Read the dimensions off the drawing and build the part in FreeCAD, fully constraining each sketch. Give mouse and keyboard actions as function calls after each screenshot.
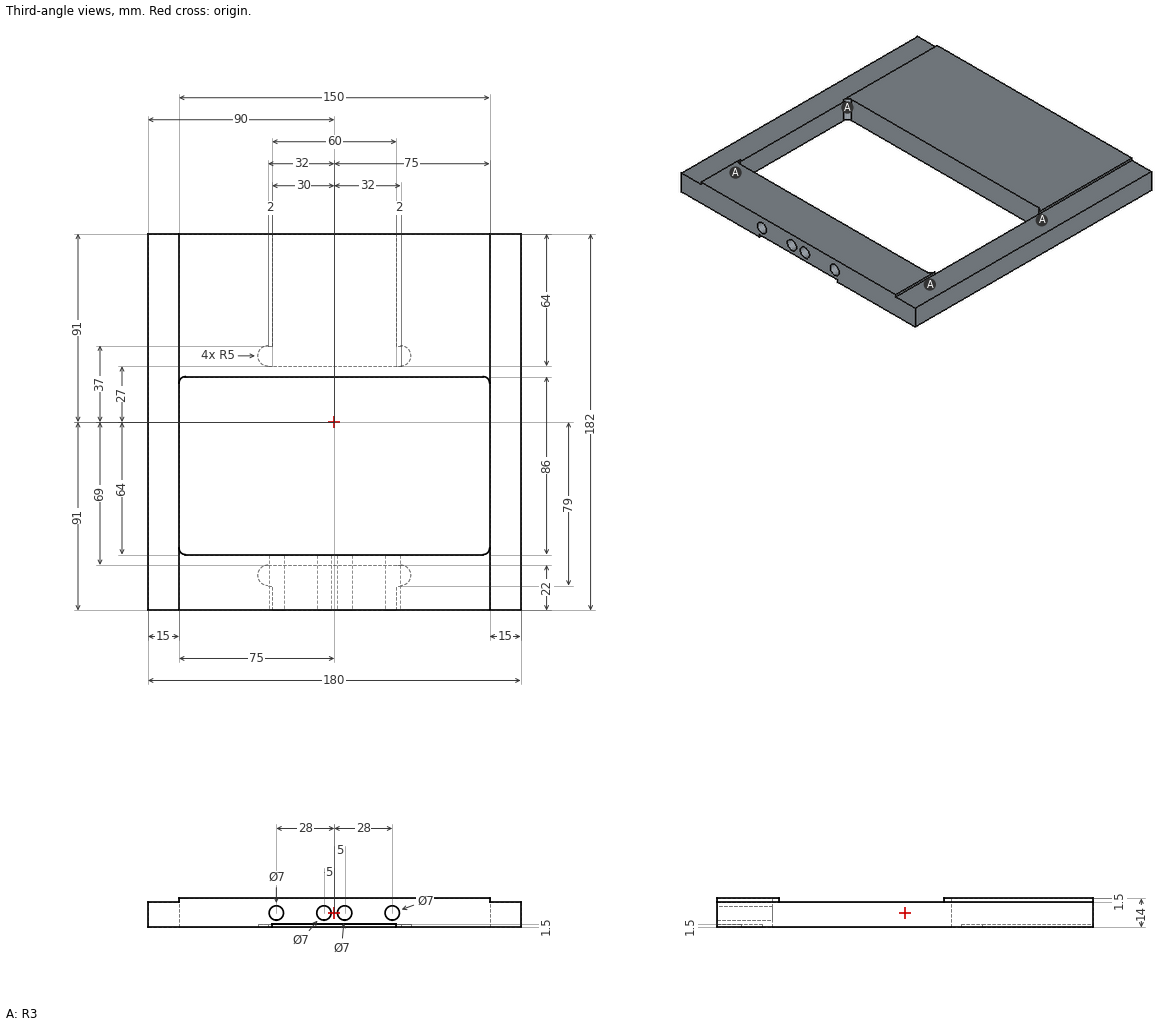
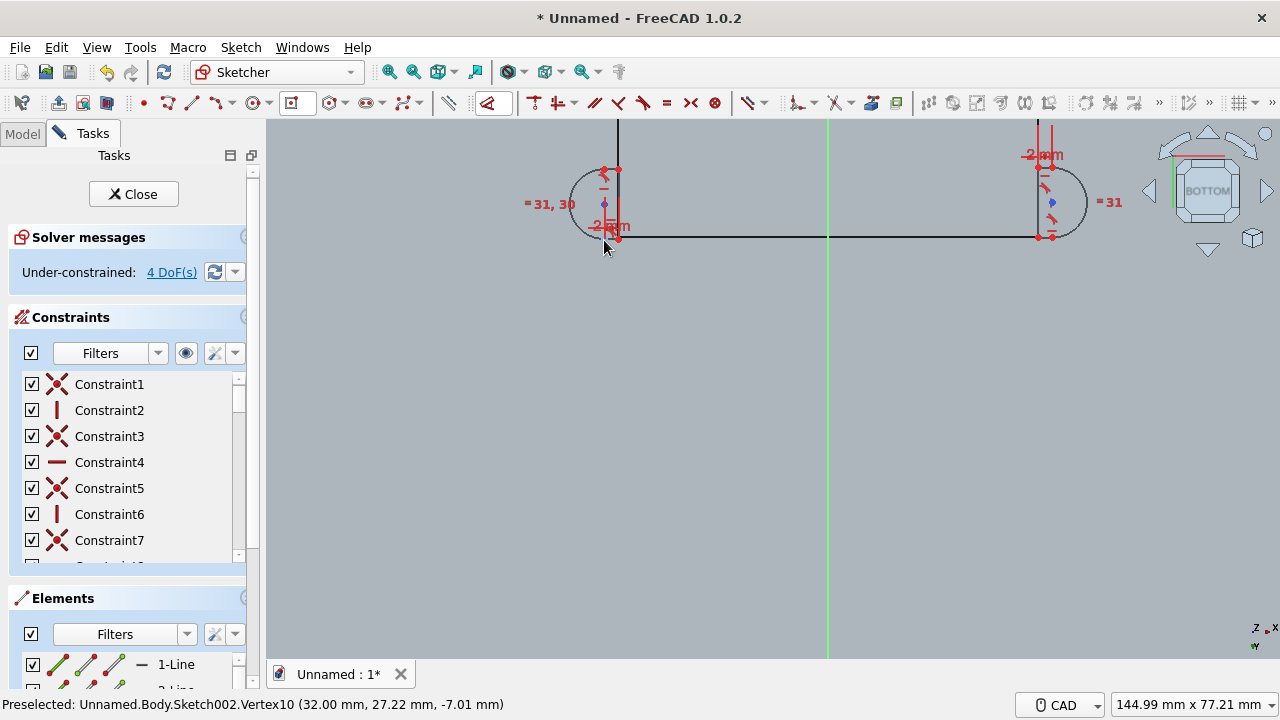
click(605, 239)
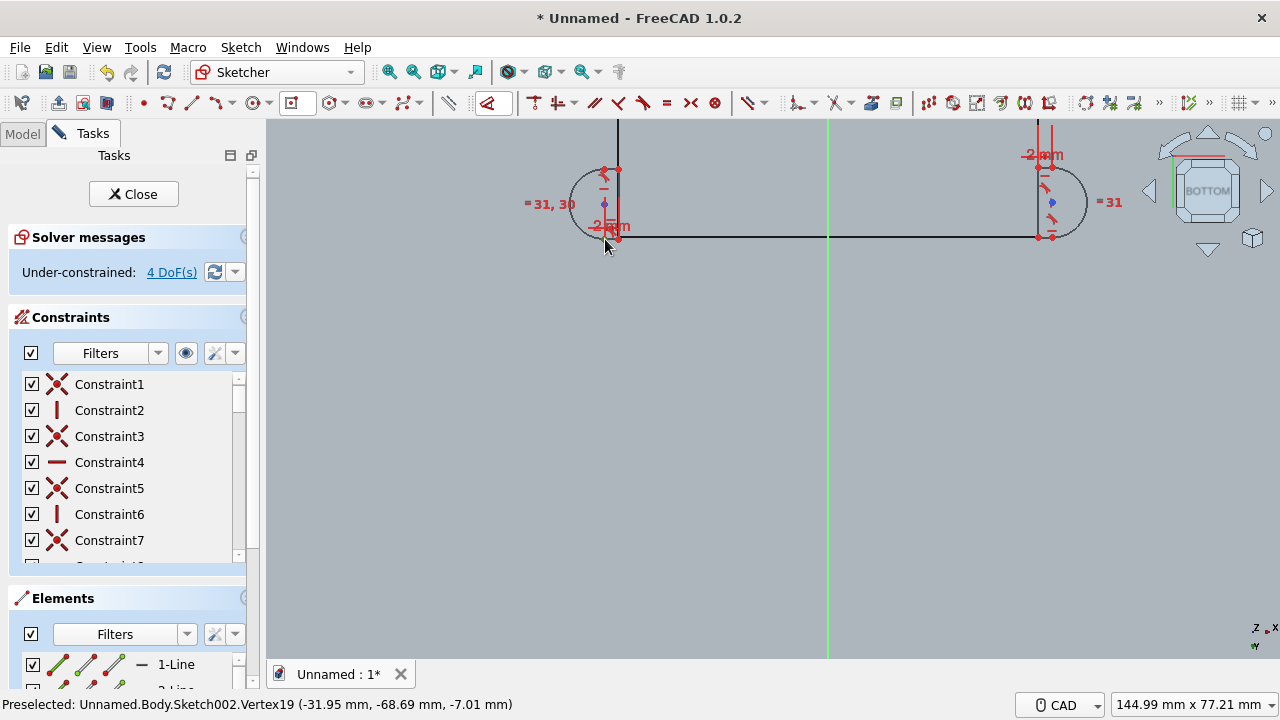
key(l)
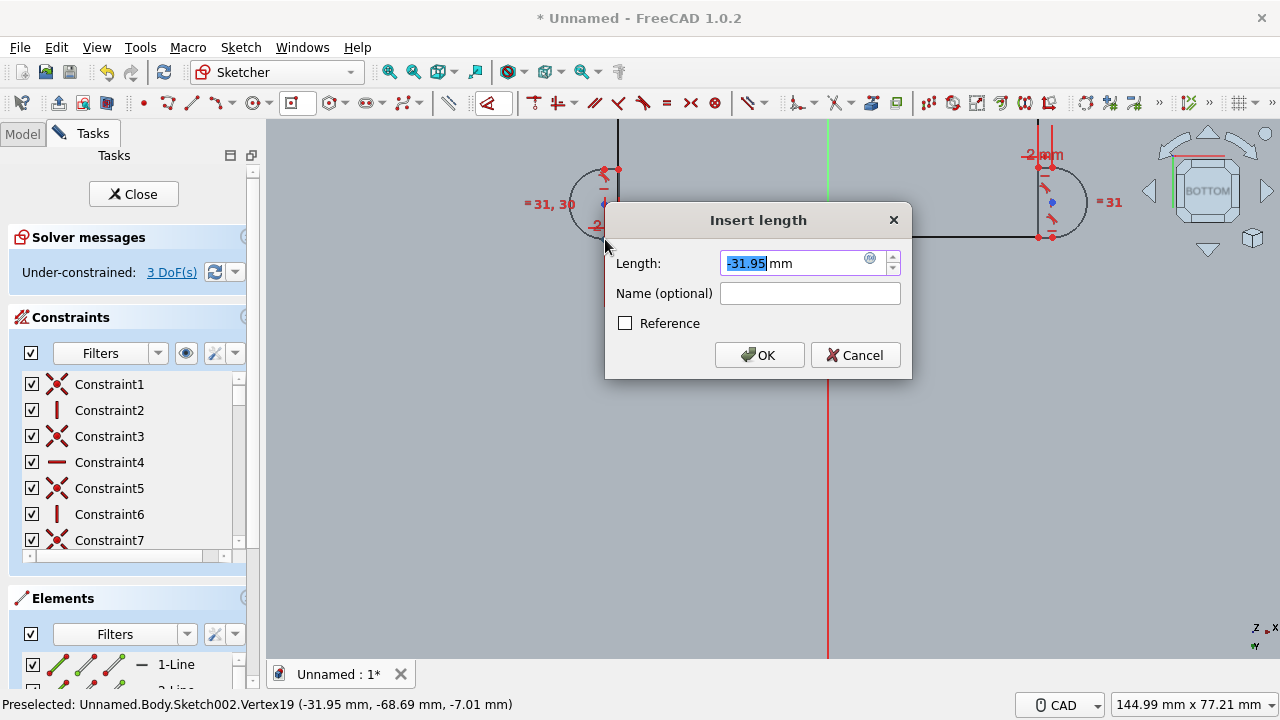
text(-32)
key(Return)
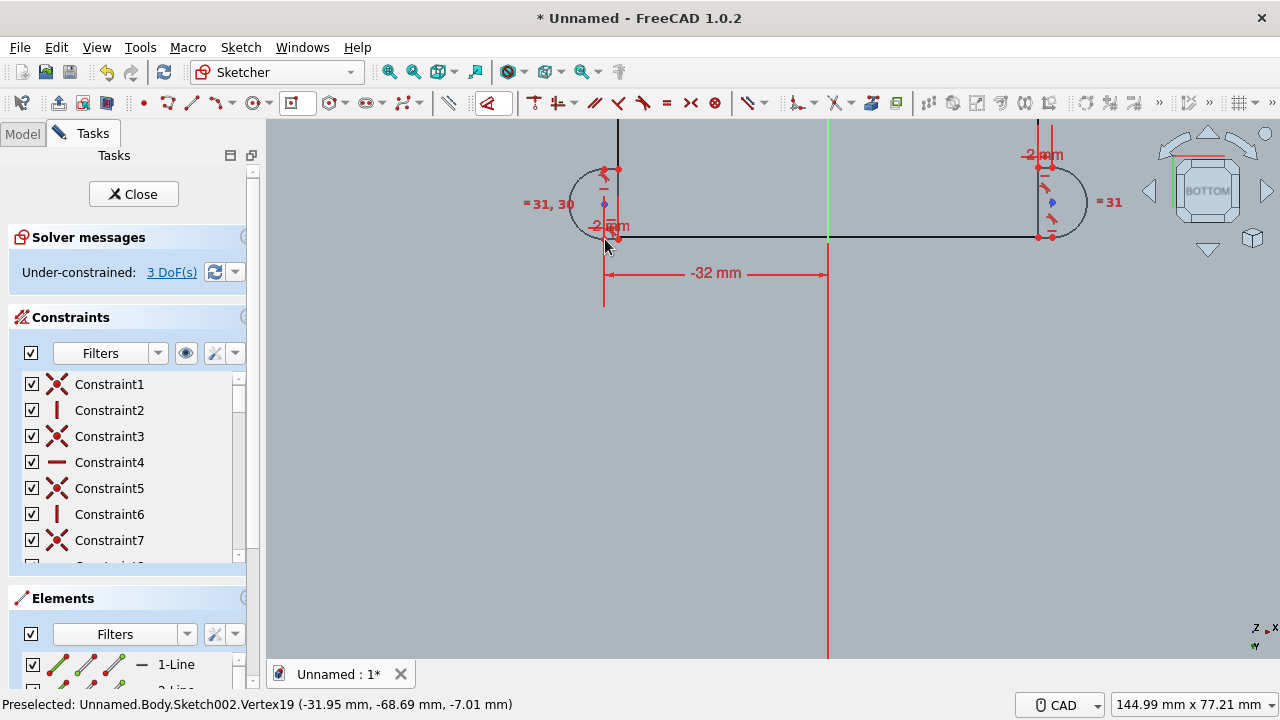
click(604, 239)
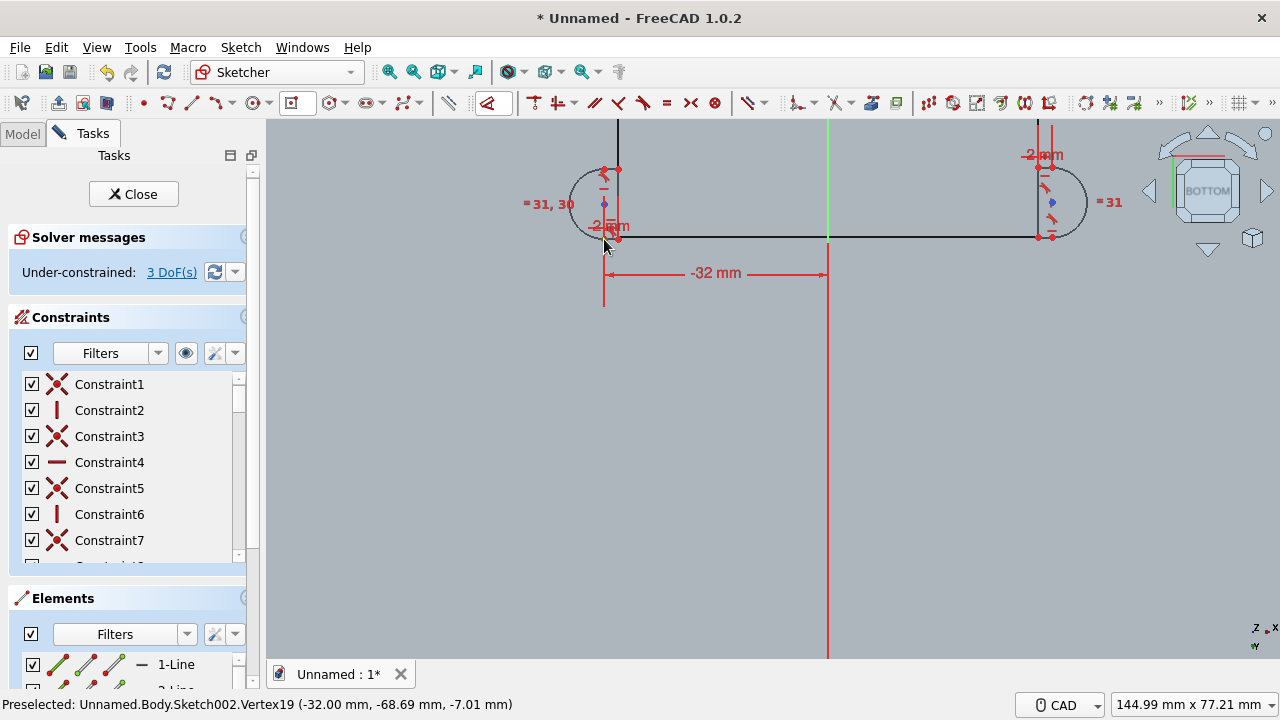
click(506, 104)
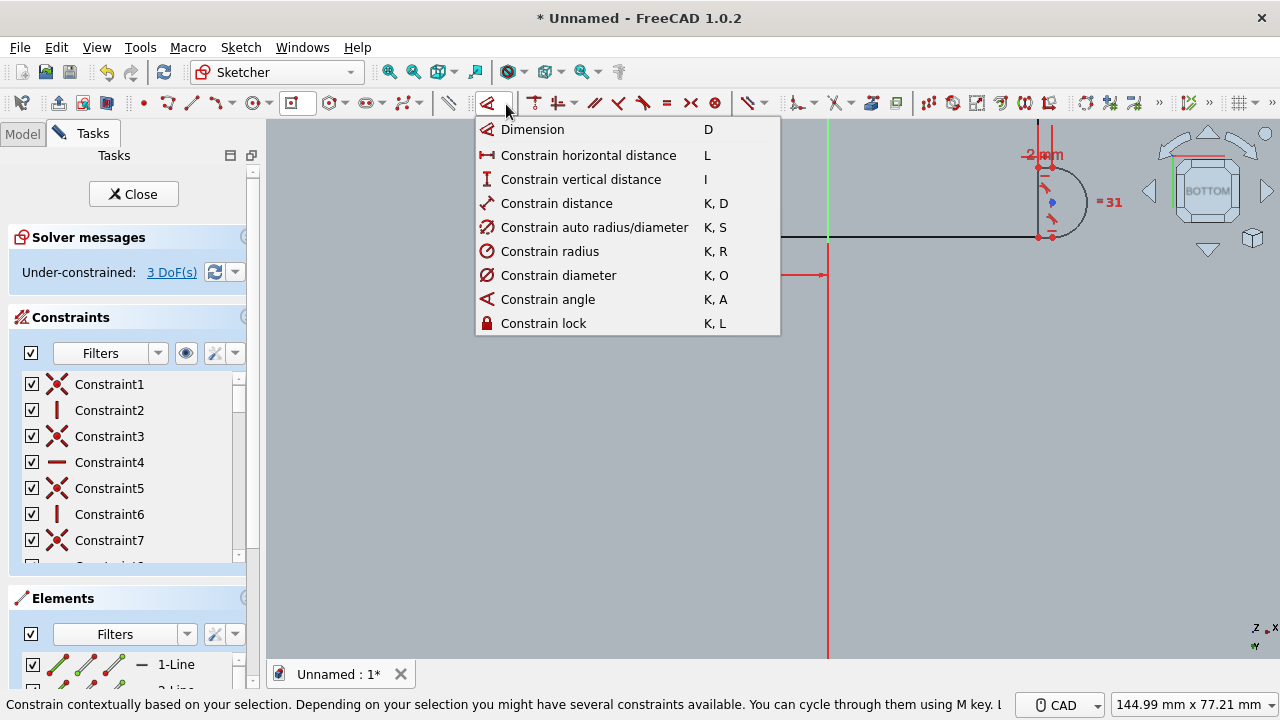
click(628, 179)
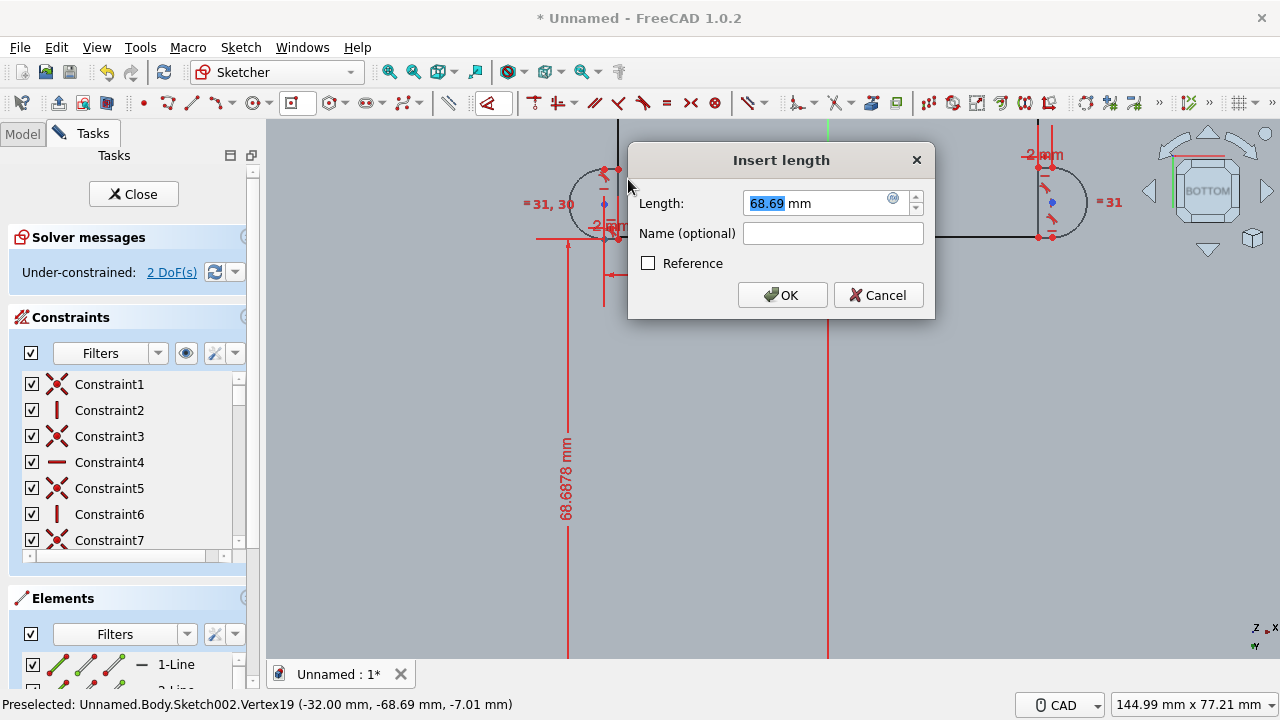
text(69)
key(Return)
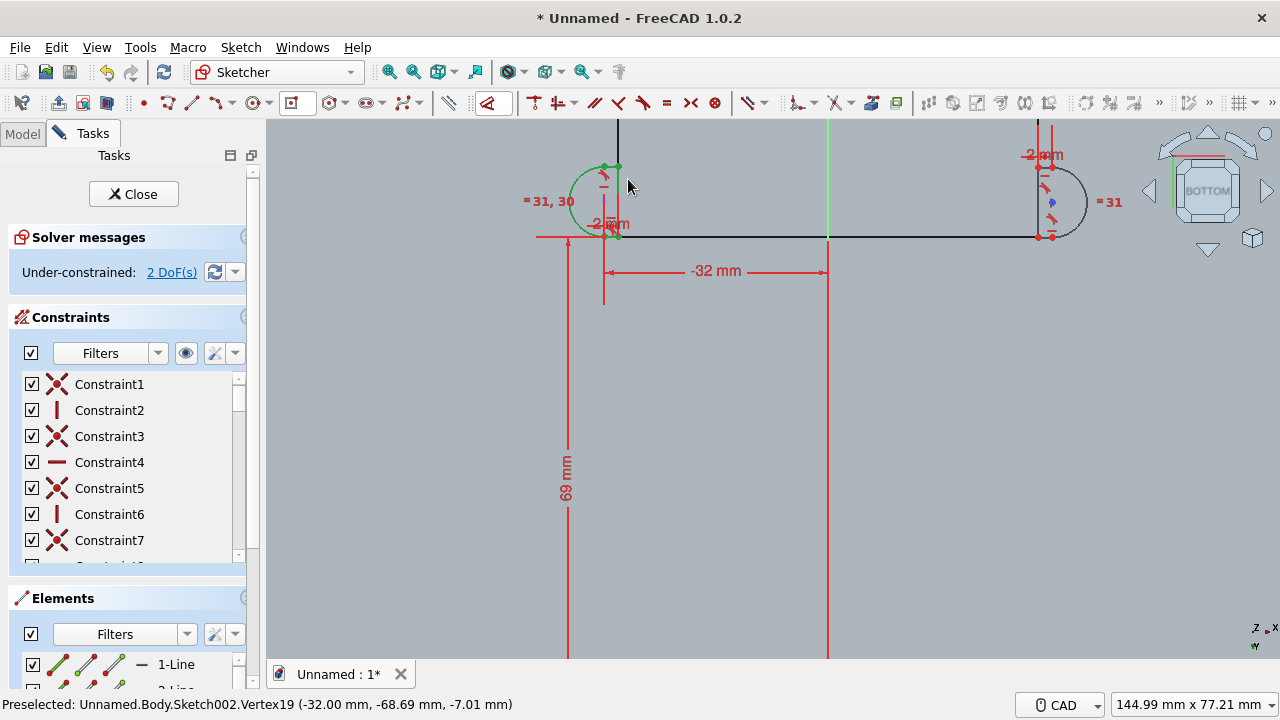
click(1052, 168)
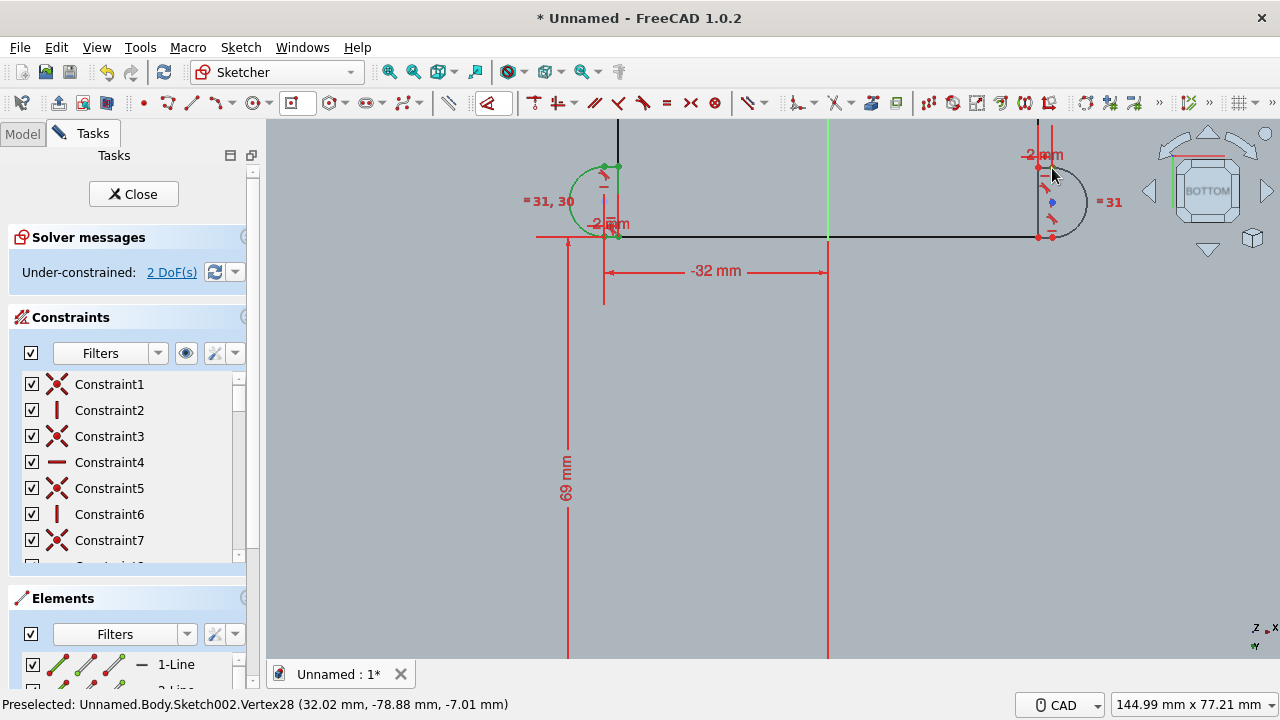
key(l)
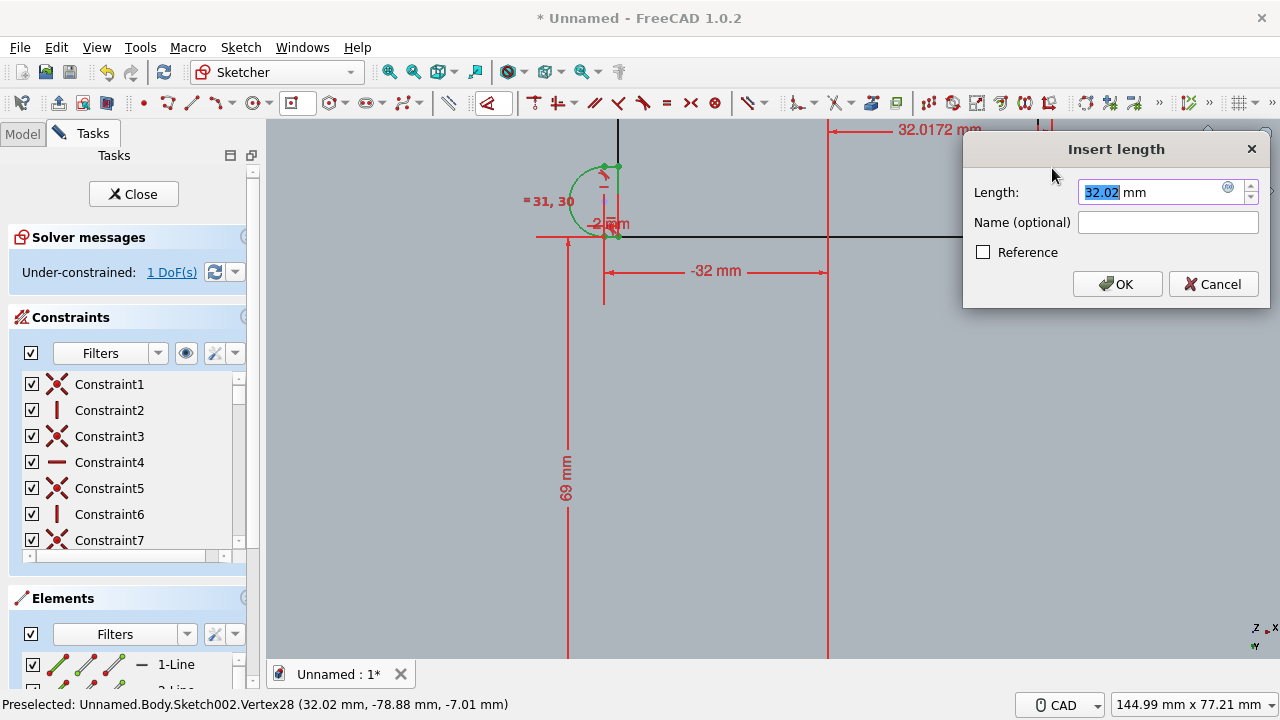
text(32)
key(Return)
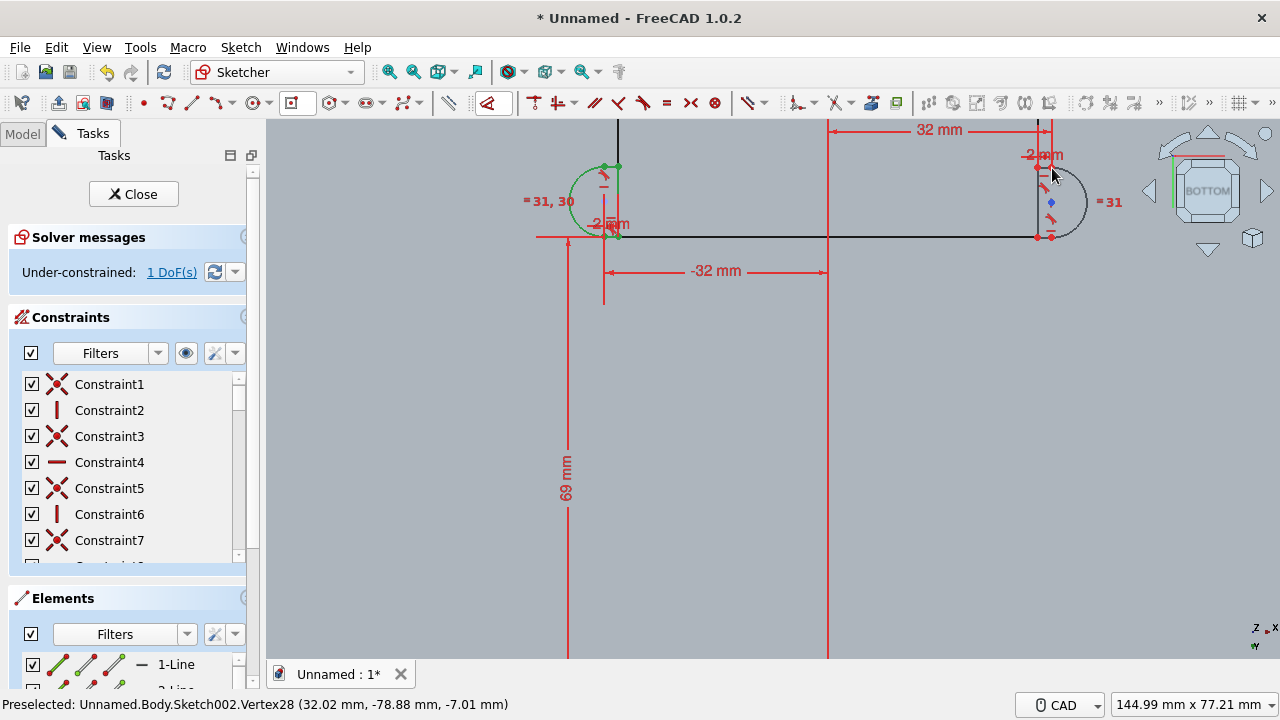
click(1052, 168)